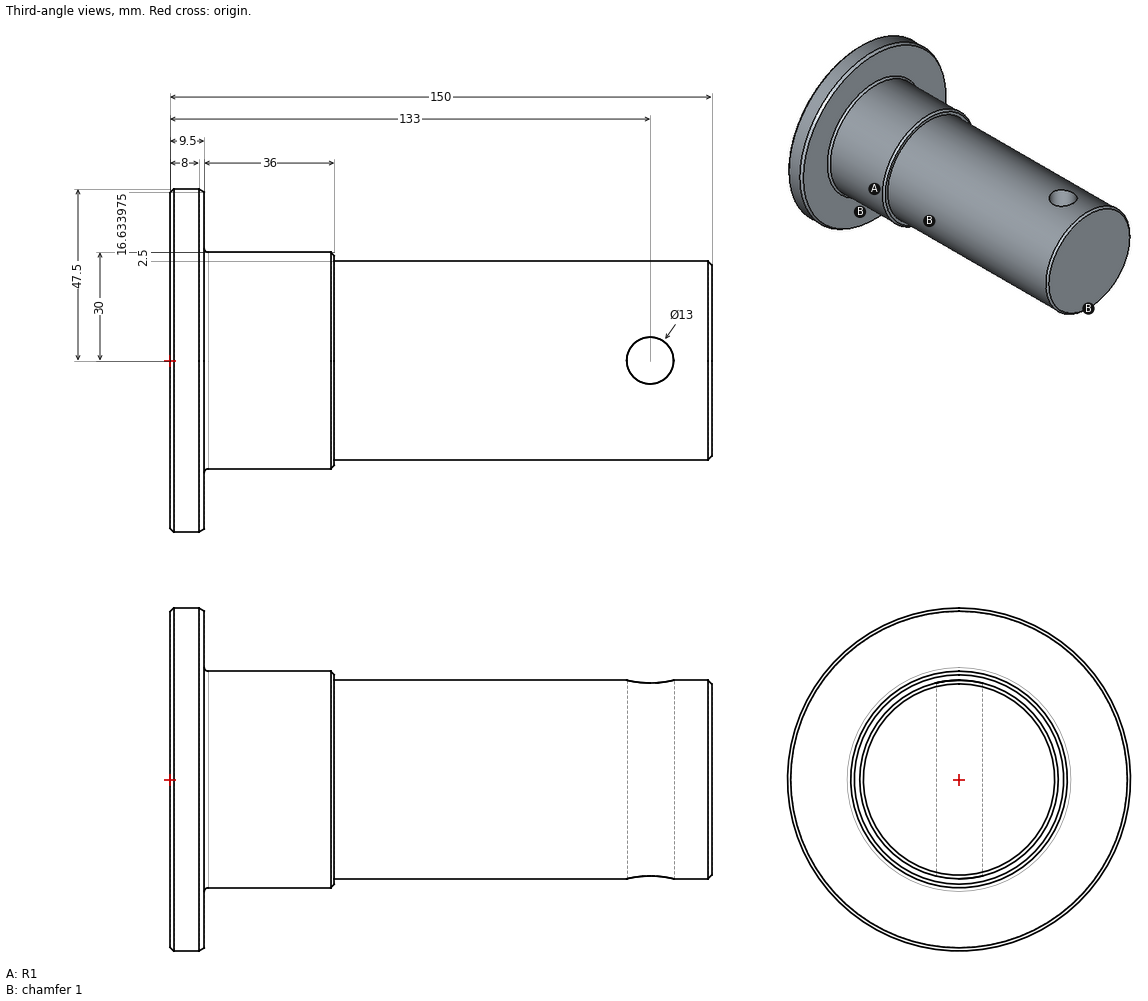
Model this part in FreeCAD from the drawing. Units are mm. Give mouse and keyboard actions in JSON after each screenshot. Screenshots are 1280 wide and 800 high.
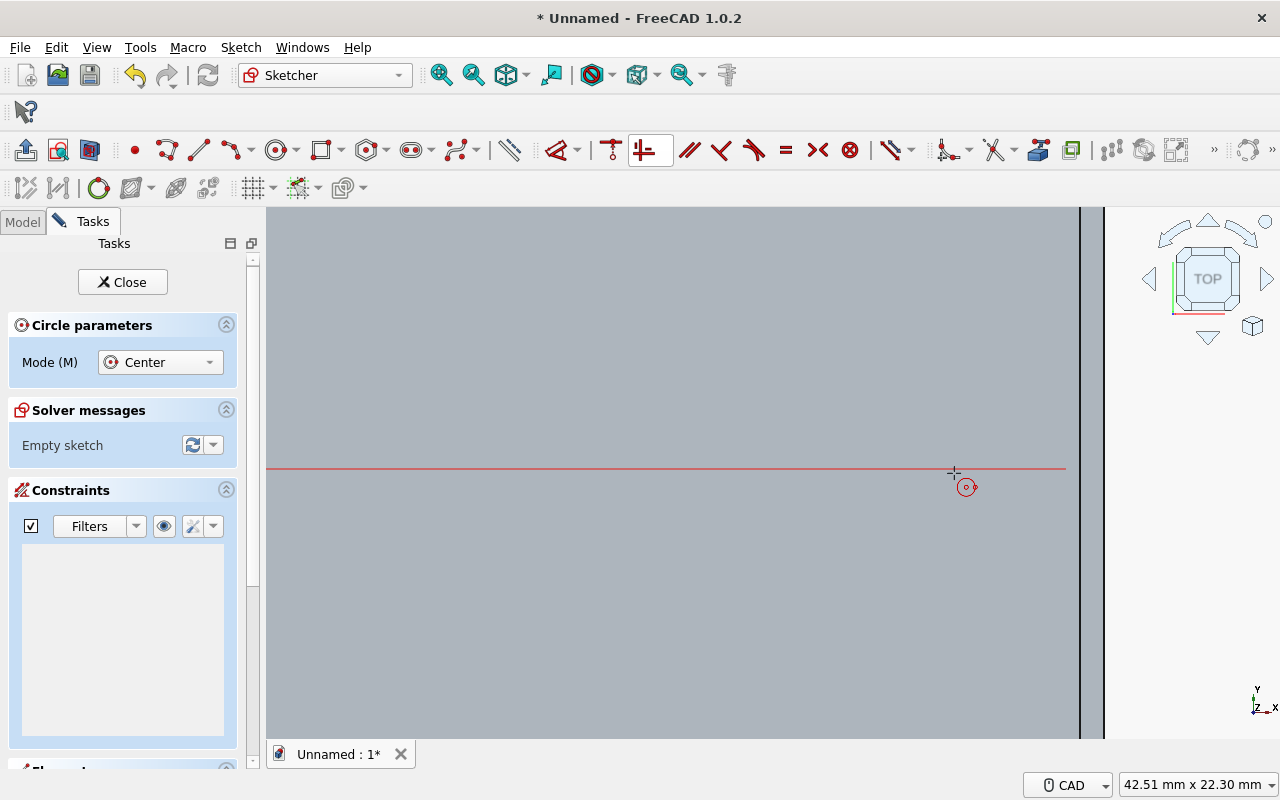
{"action": "left_click", "coordinate": [699, 469]}
{"action": "left_click", "coordinate": [808, 359]}
{"action": "key", "text": "Escape"}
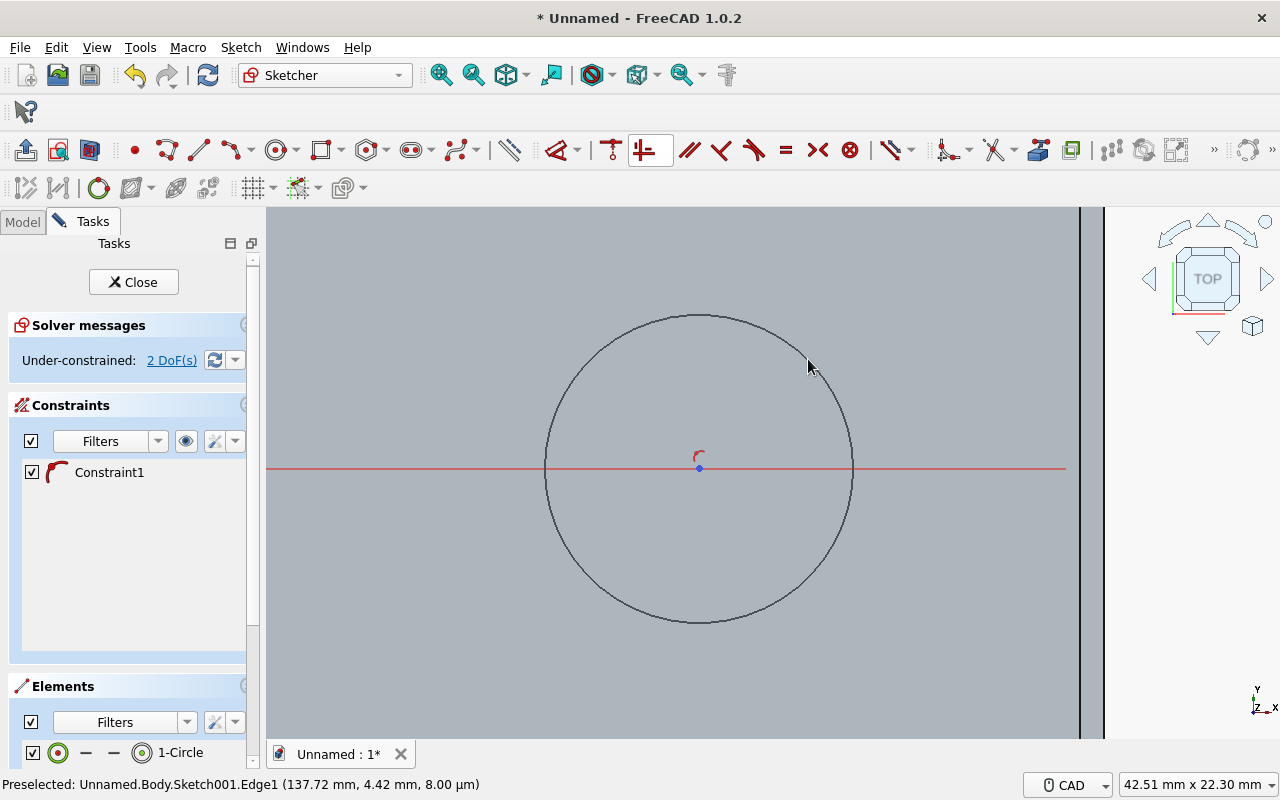
{"action": "key", "text": "d"}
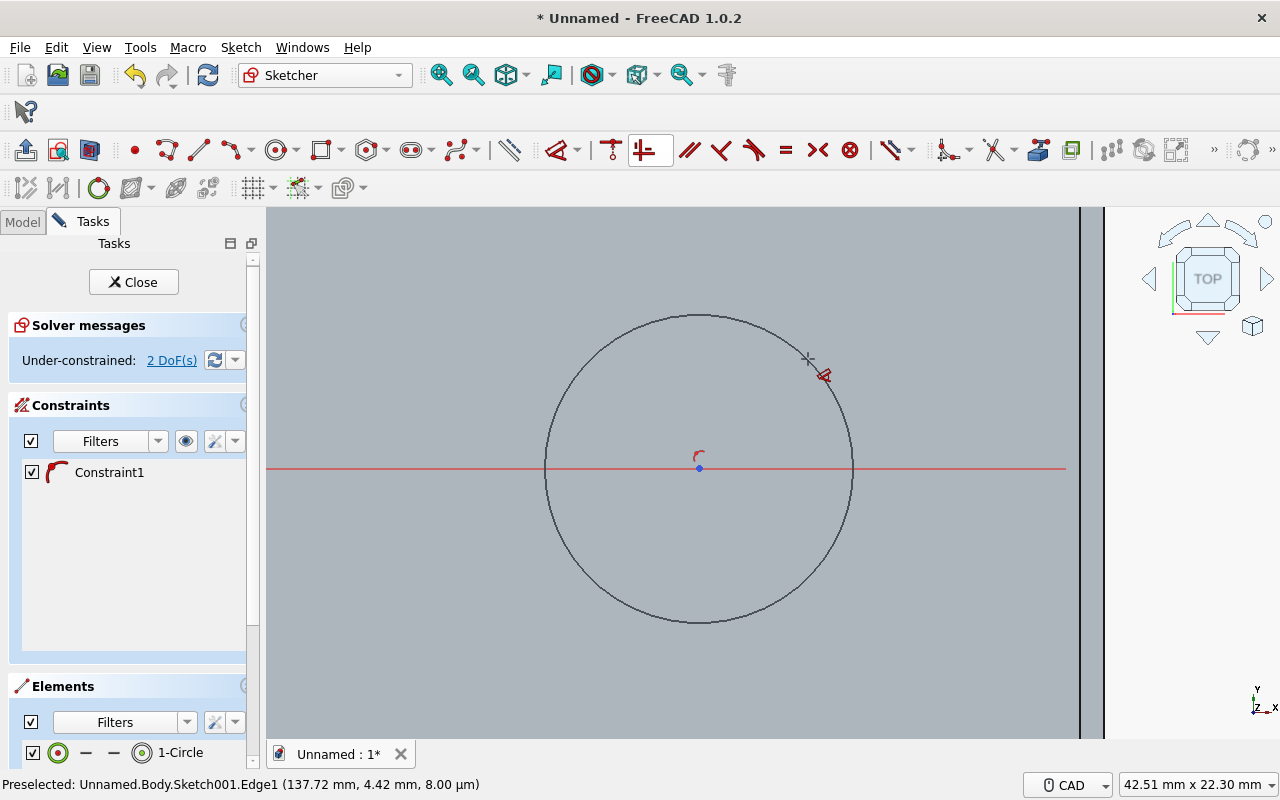
{"action": "left_click", "coordinate": [808, 360]}
{"action": "left_click", "coordinate": [831, 337]}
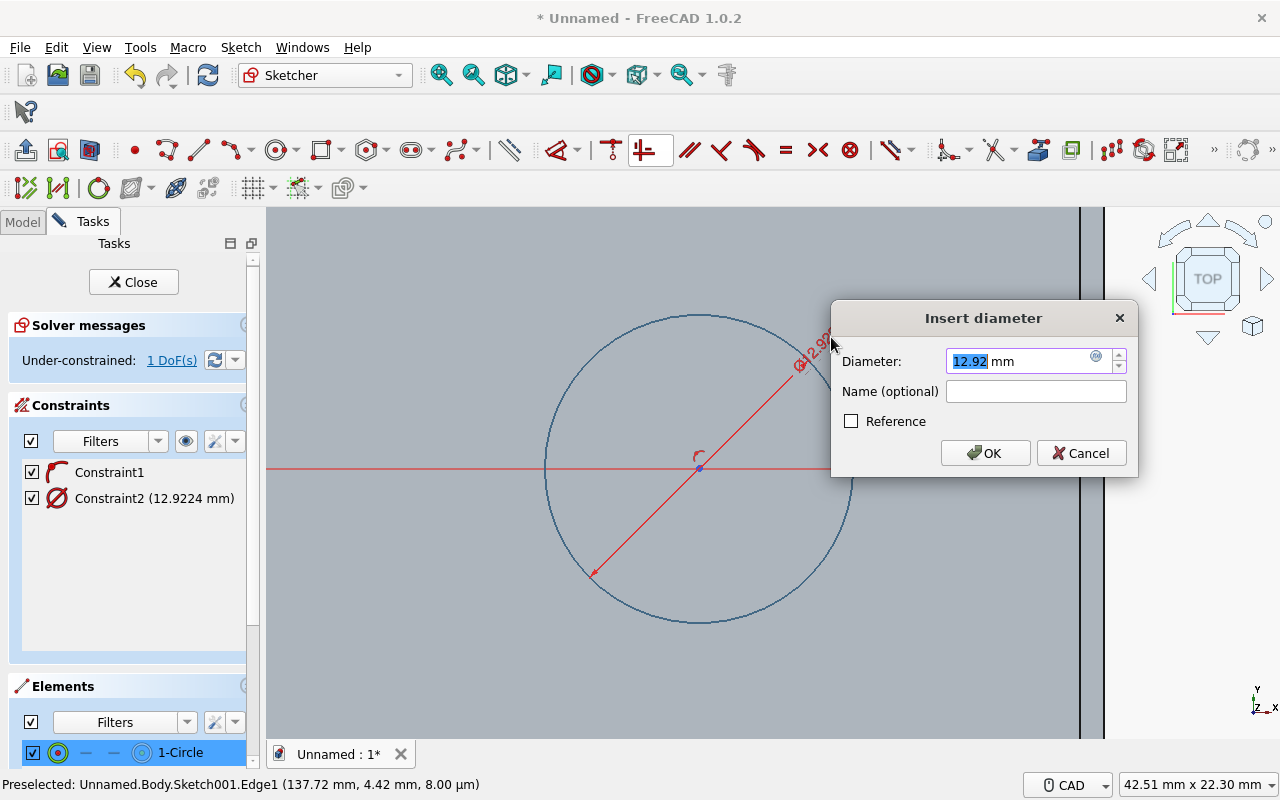
{"action": "type", "text": "13"}
{"action": "key", "text": "Return"}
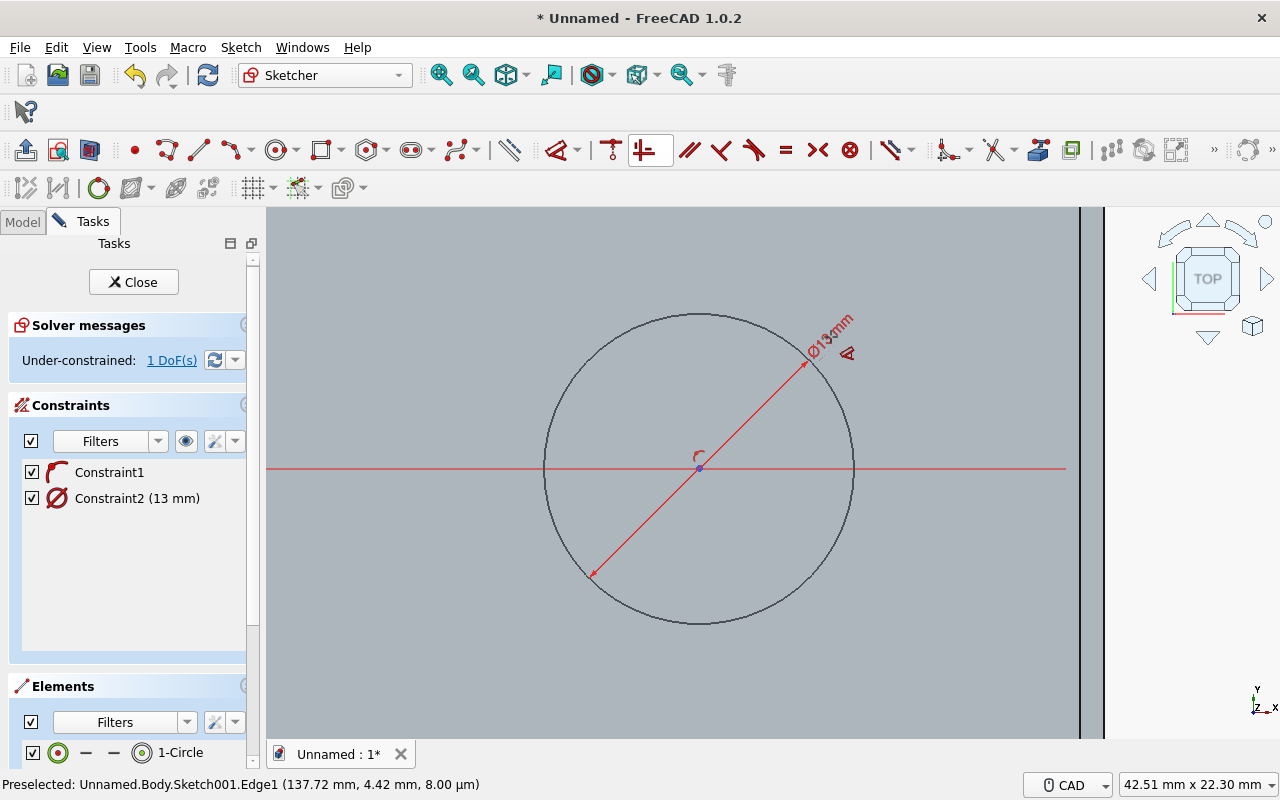
{"action": "left_click", "coordinate": [699, 469]}
{"action": "left_click", "coordinate": [497, 503]}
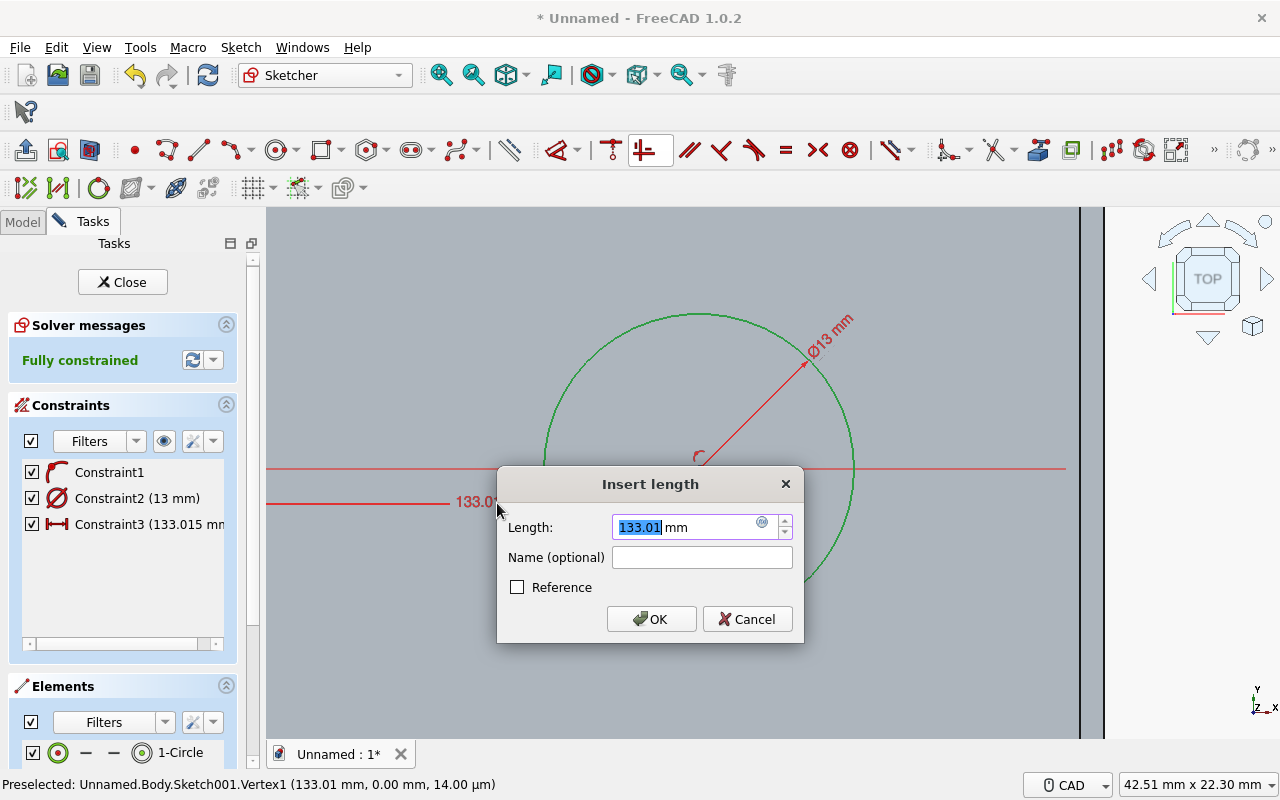
{"action": "type", "text": "133"}
{"action": "key", "text": "Return"}
{"action": "key", "text": "Escape"}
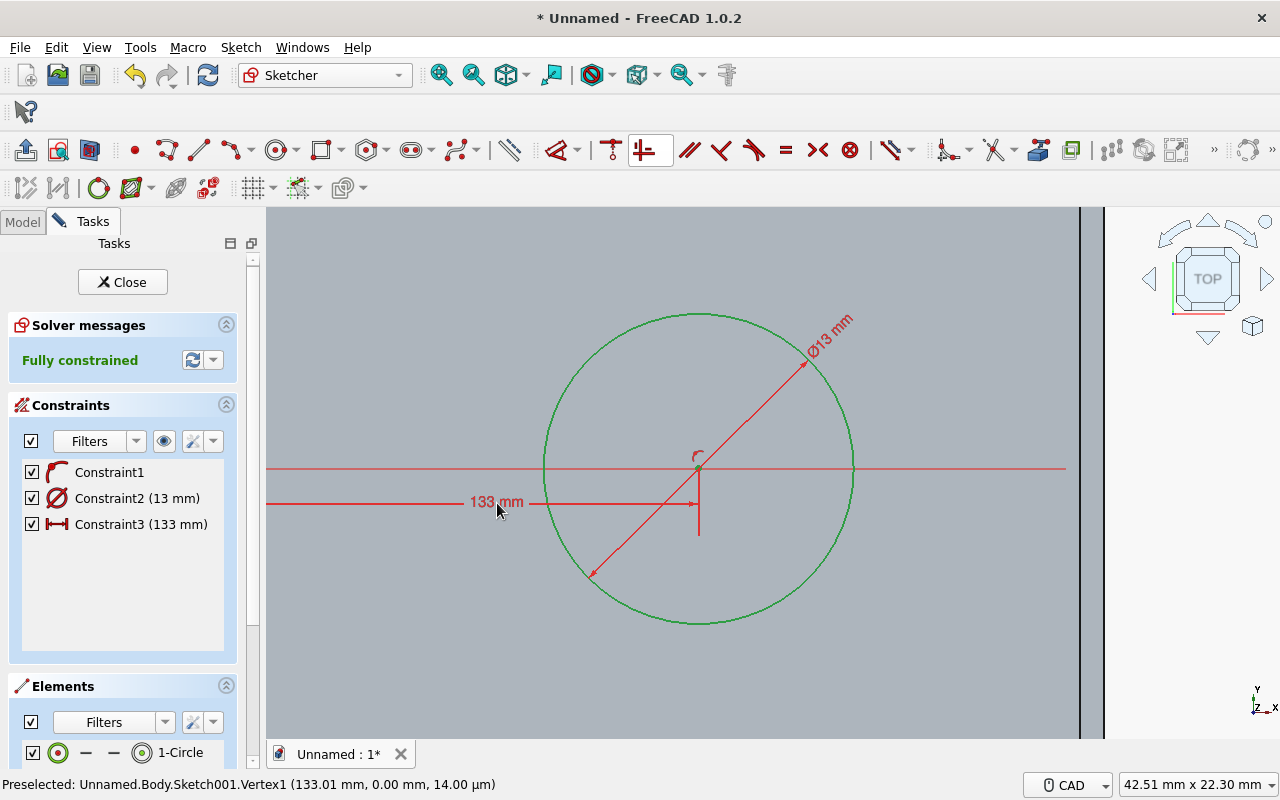
{"action": "left_click", "coordinate": [123, 282]}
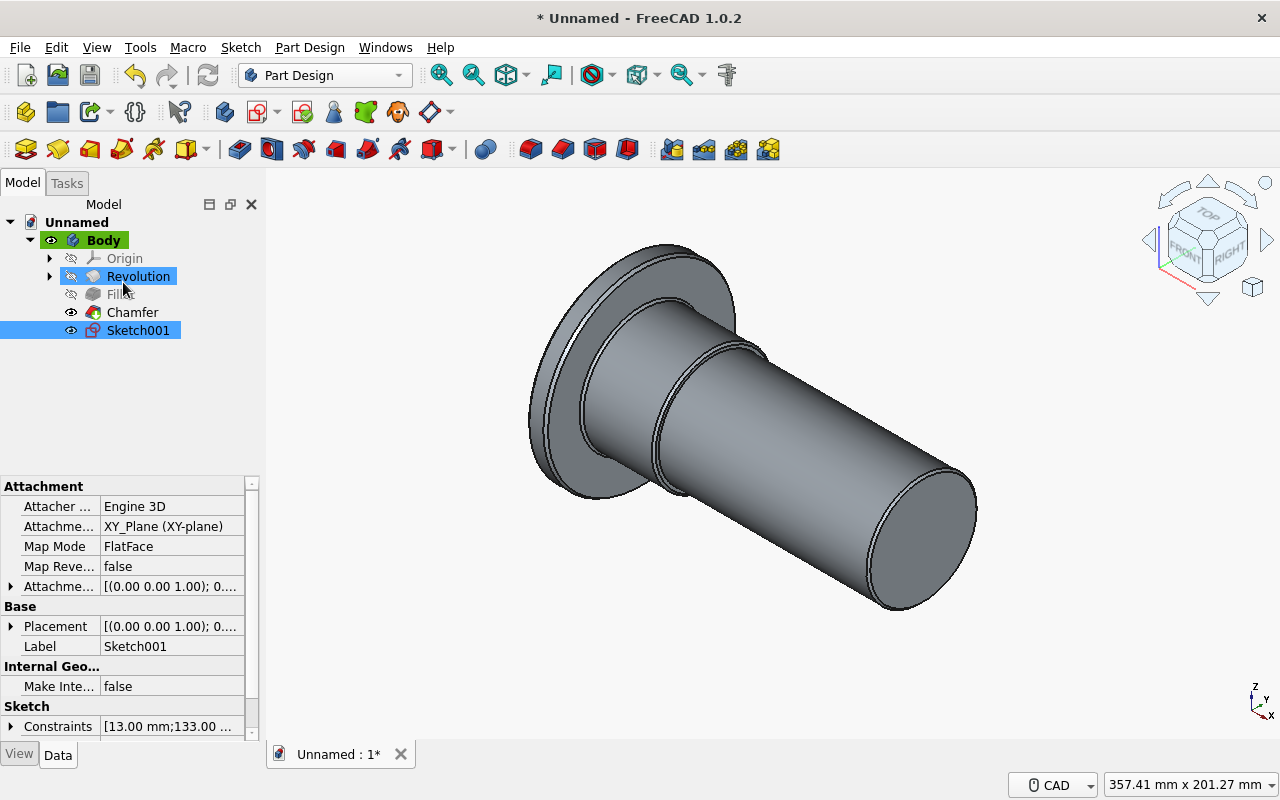
{"action": "left_click", "coordinate": [240, 150]}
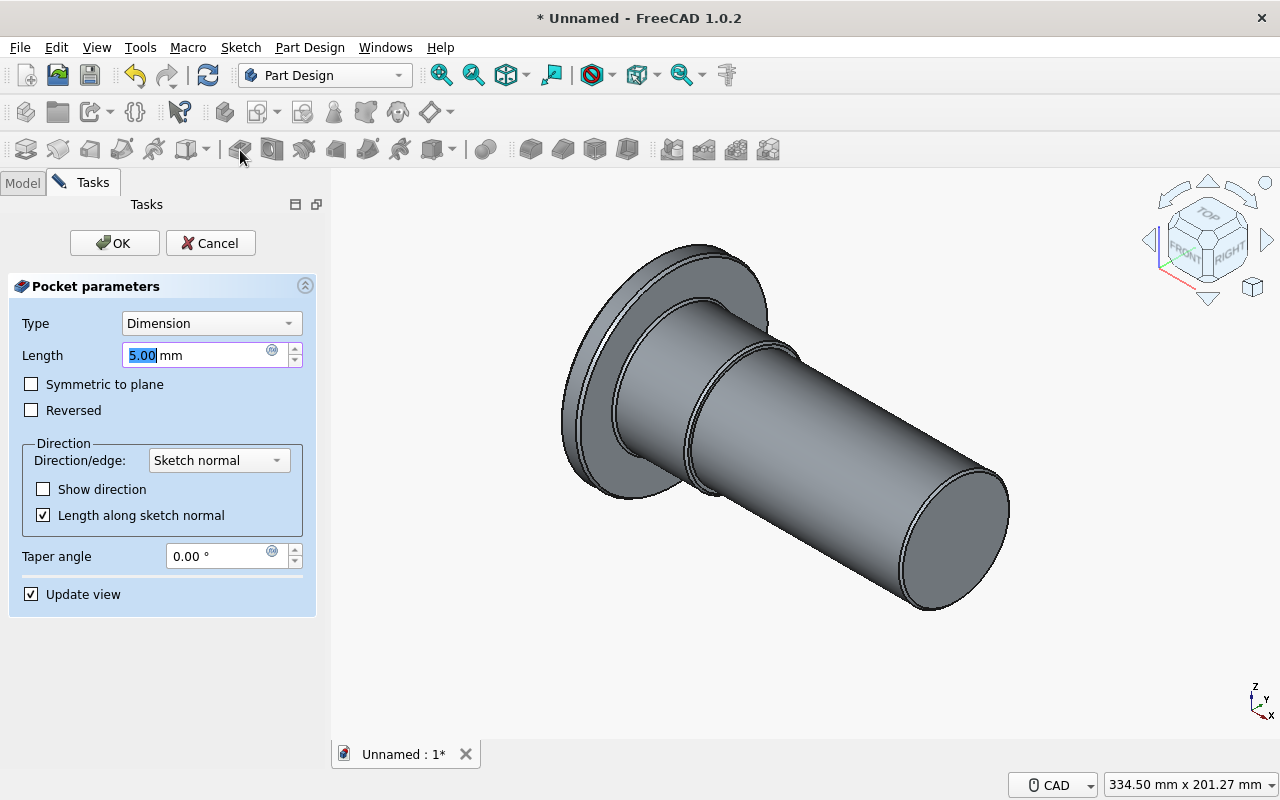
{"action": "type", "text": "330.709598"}
{"action": "key", "text": "Tab"}